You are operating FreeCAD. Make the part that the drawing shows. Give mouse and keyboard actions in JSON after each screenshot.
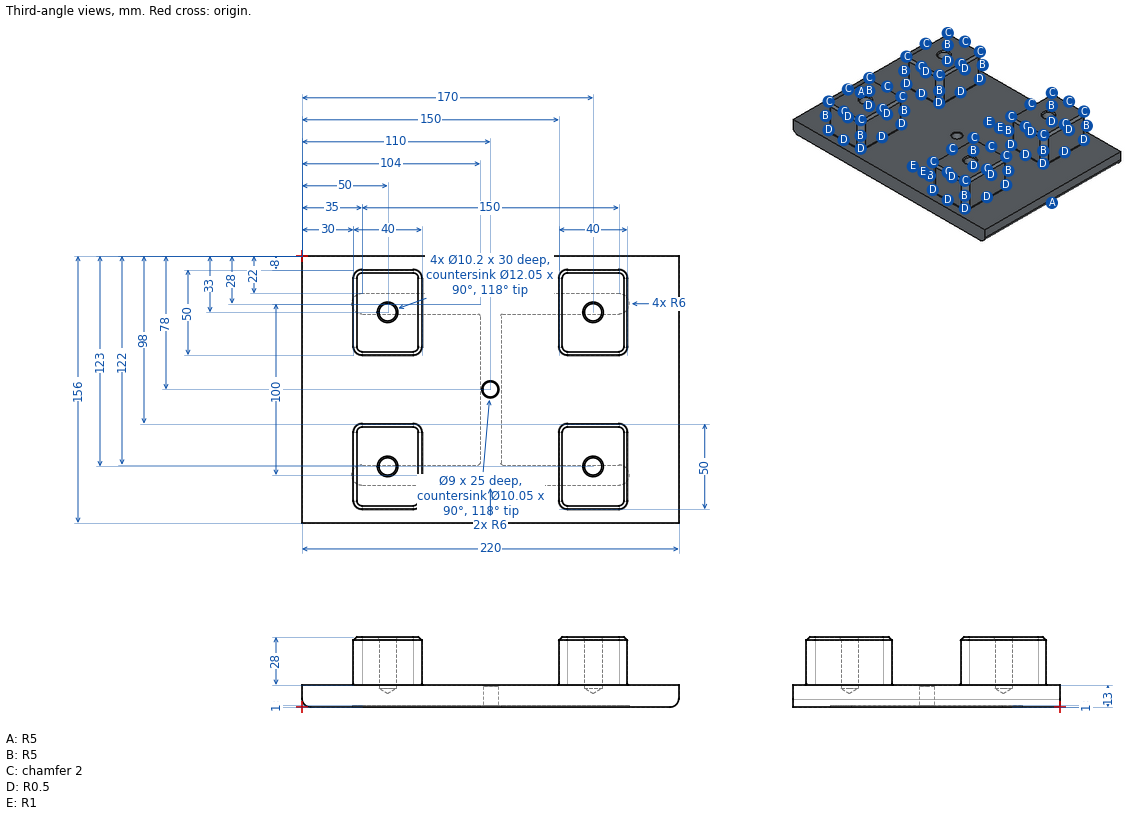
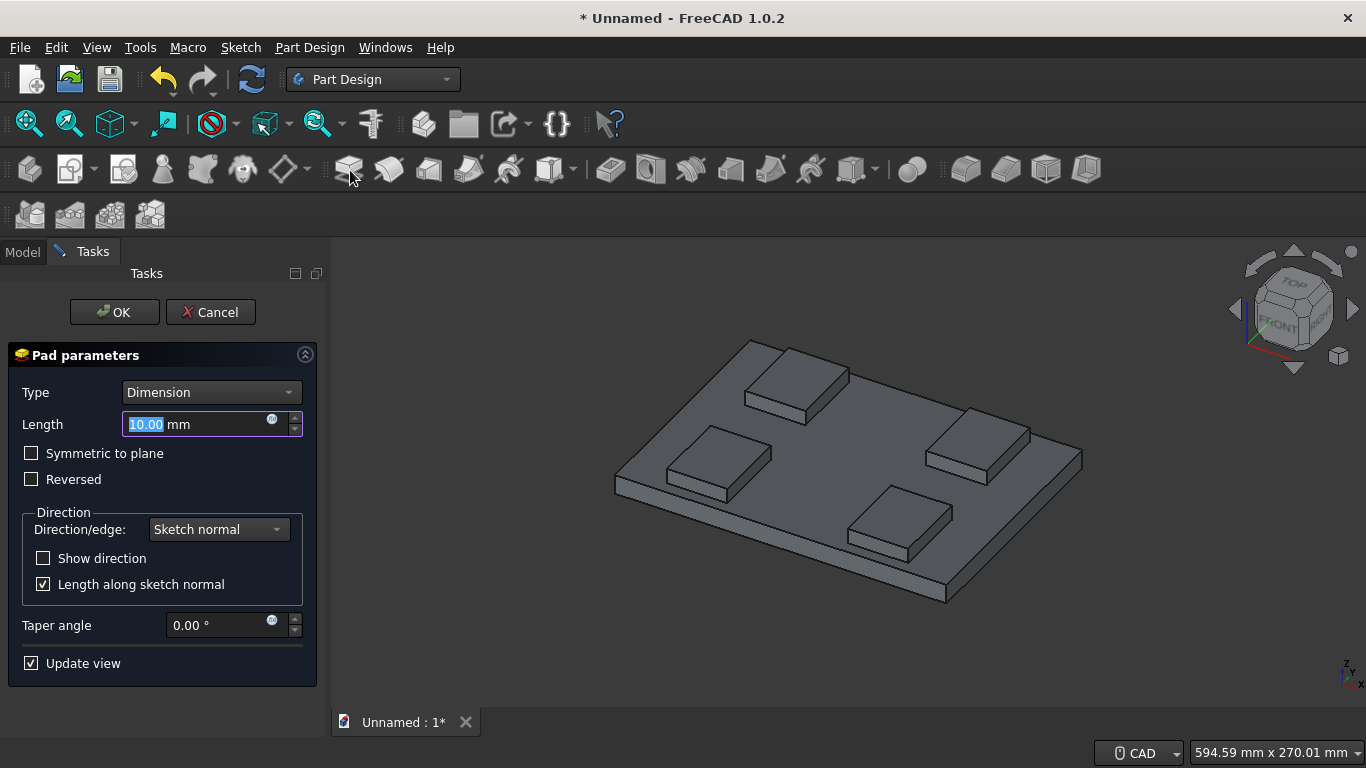
{"action": "type", "text": "28"}
{"action": "key", "text": "Tab"}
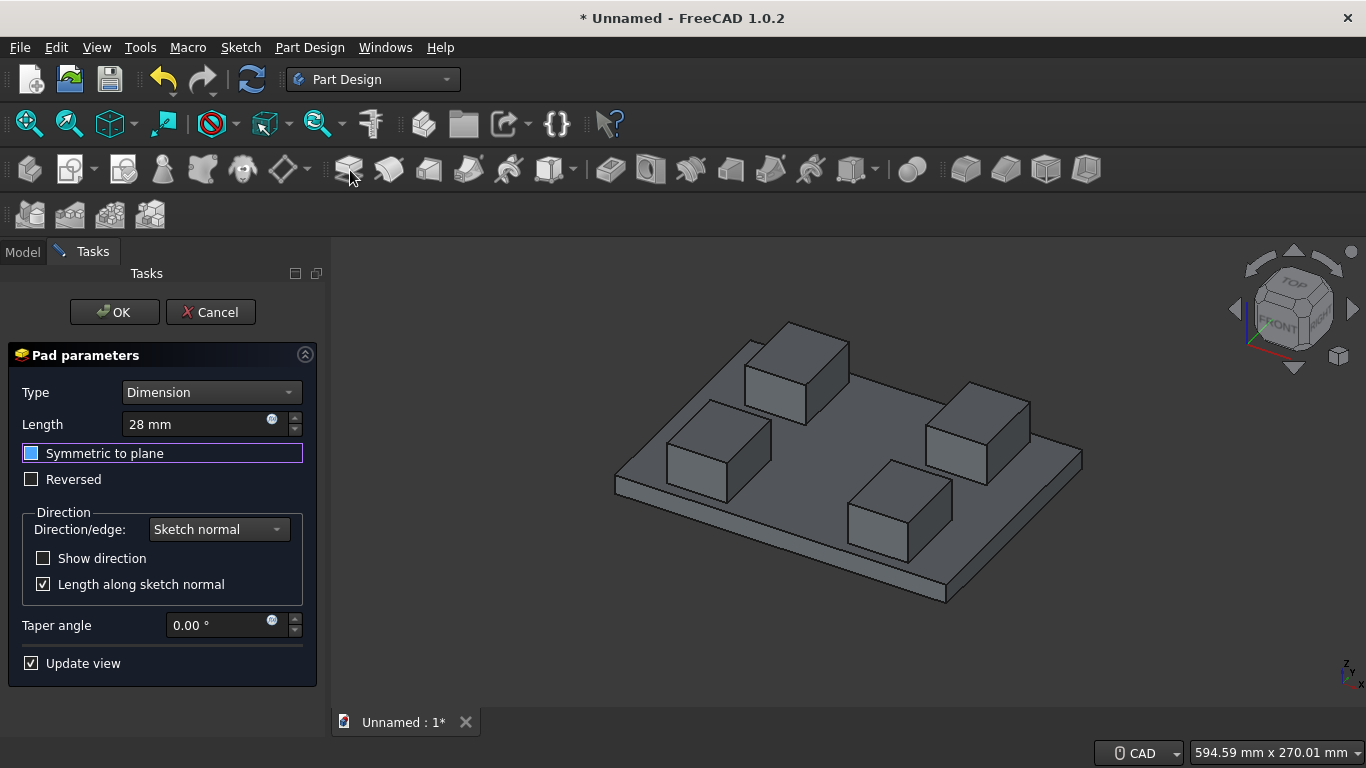
{"action": "left_click", "coordinate": [115, 312]}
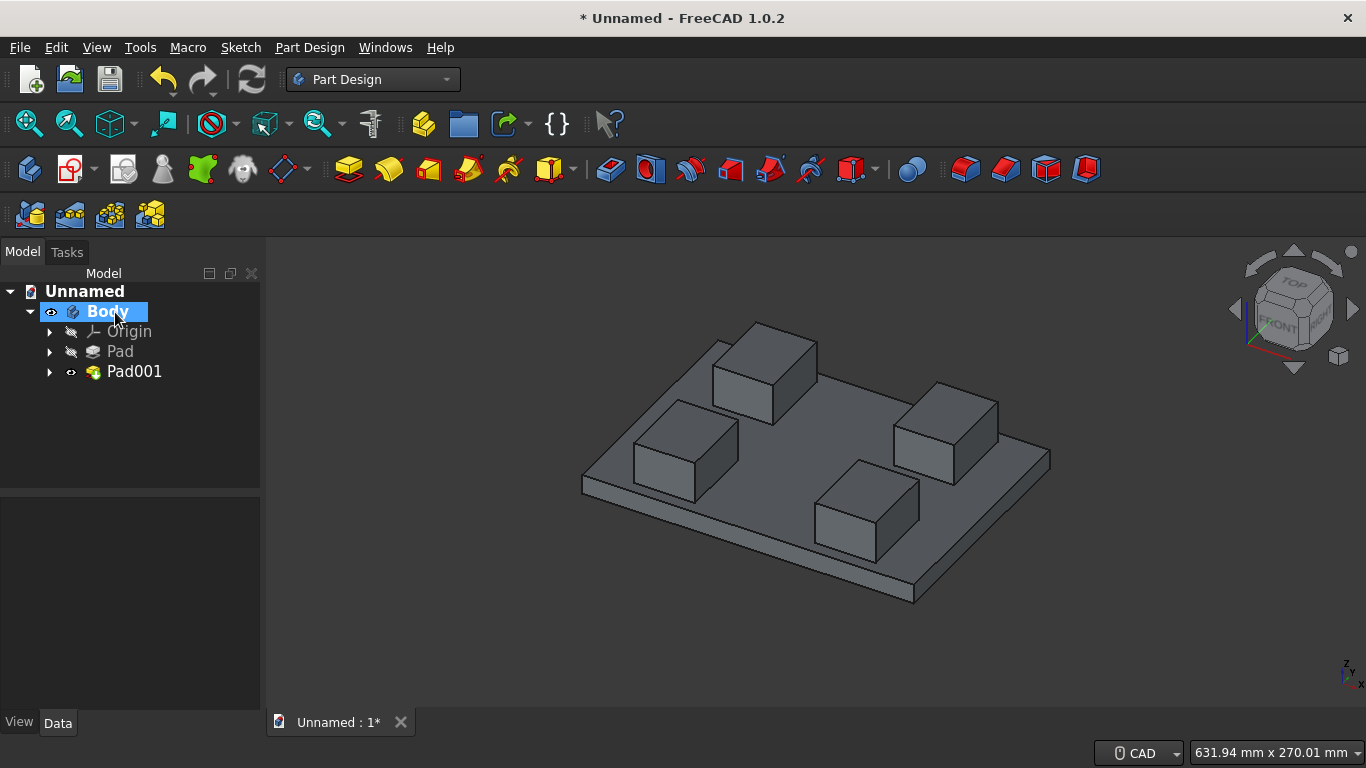
{"action": "key", "text": "0"}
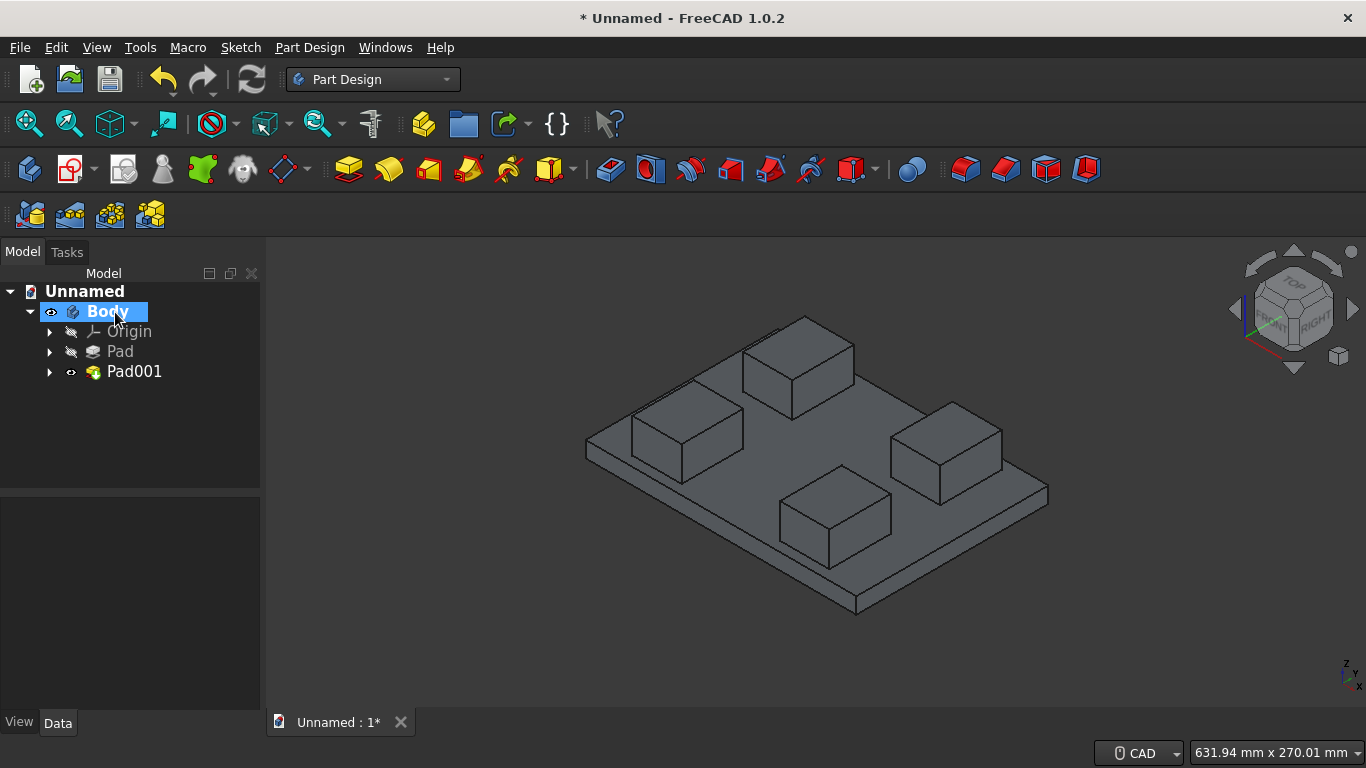
{"action": "key", "text": "2"}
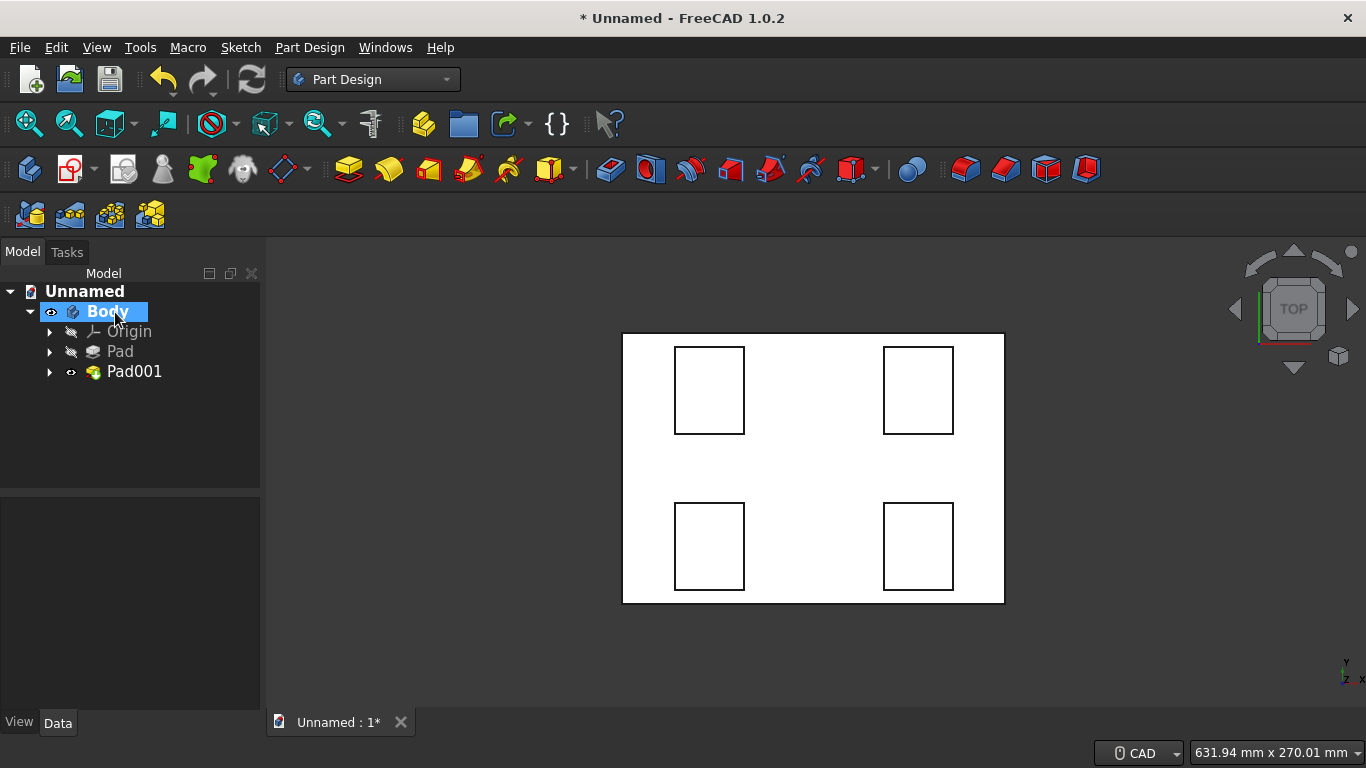
{"action": "key", "text": "1"}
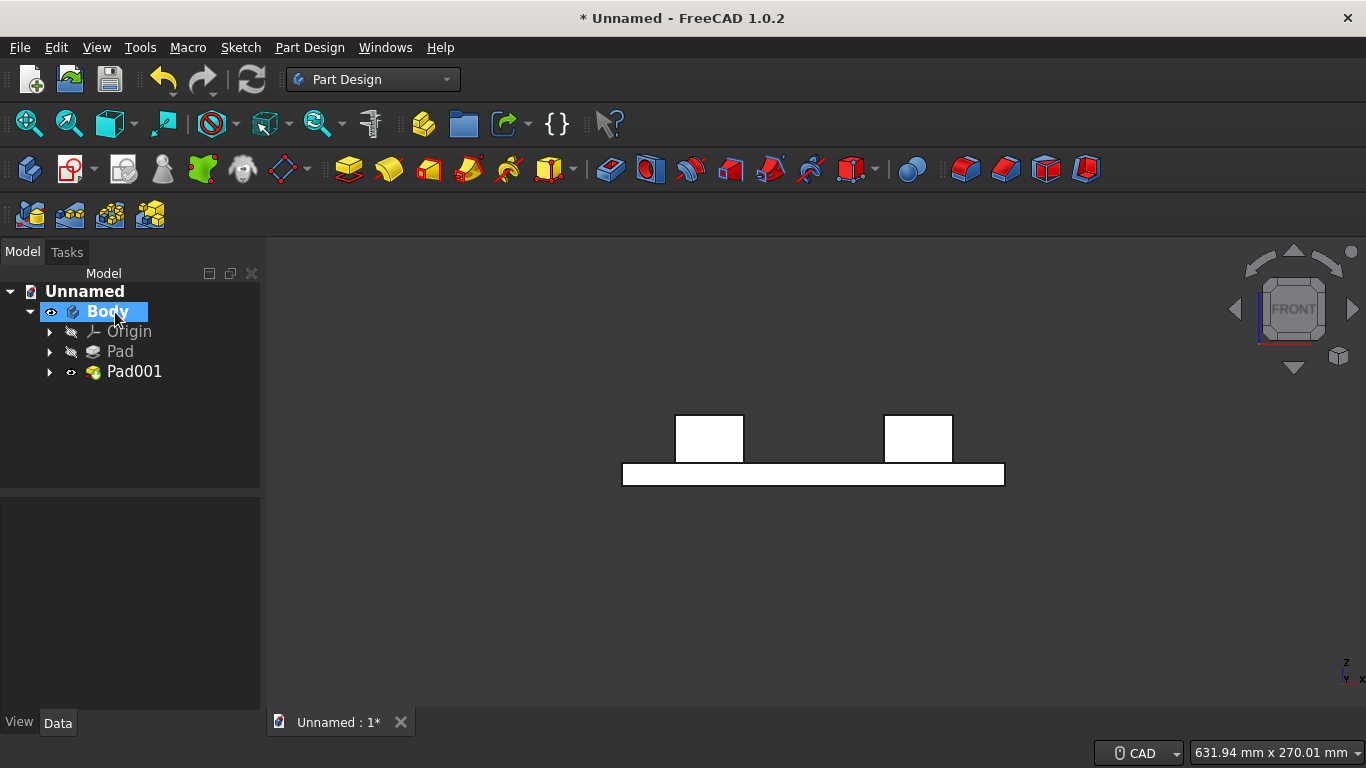
{"action": "left_click", "coordinate": [30, 124]}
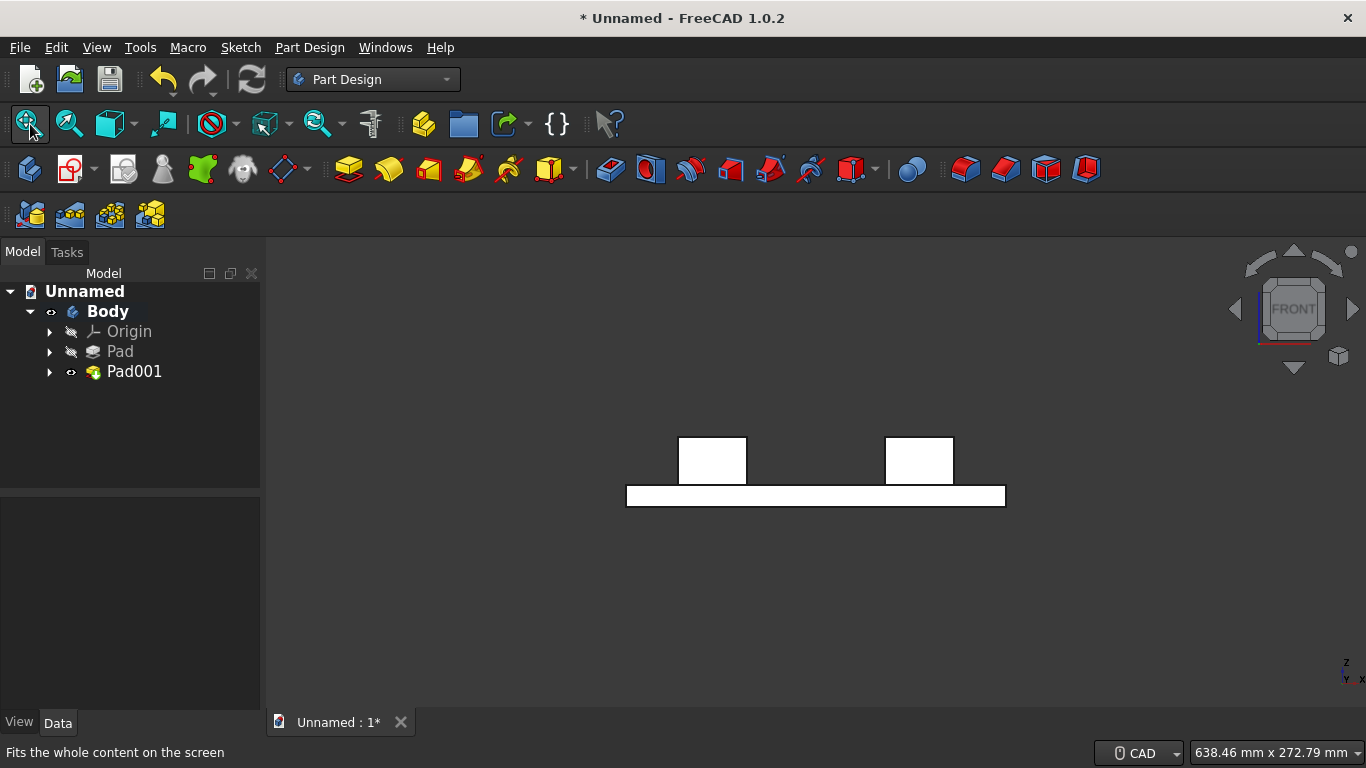
{"action": "key", "text": "3"}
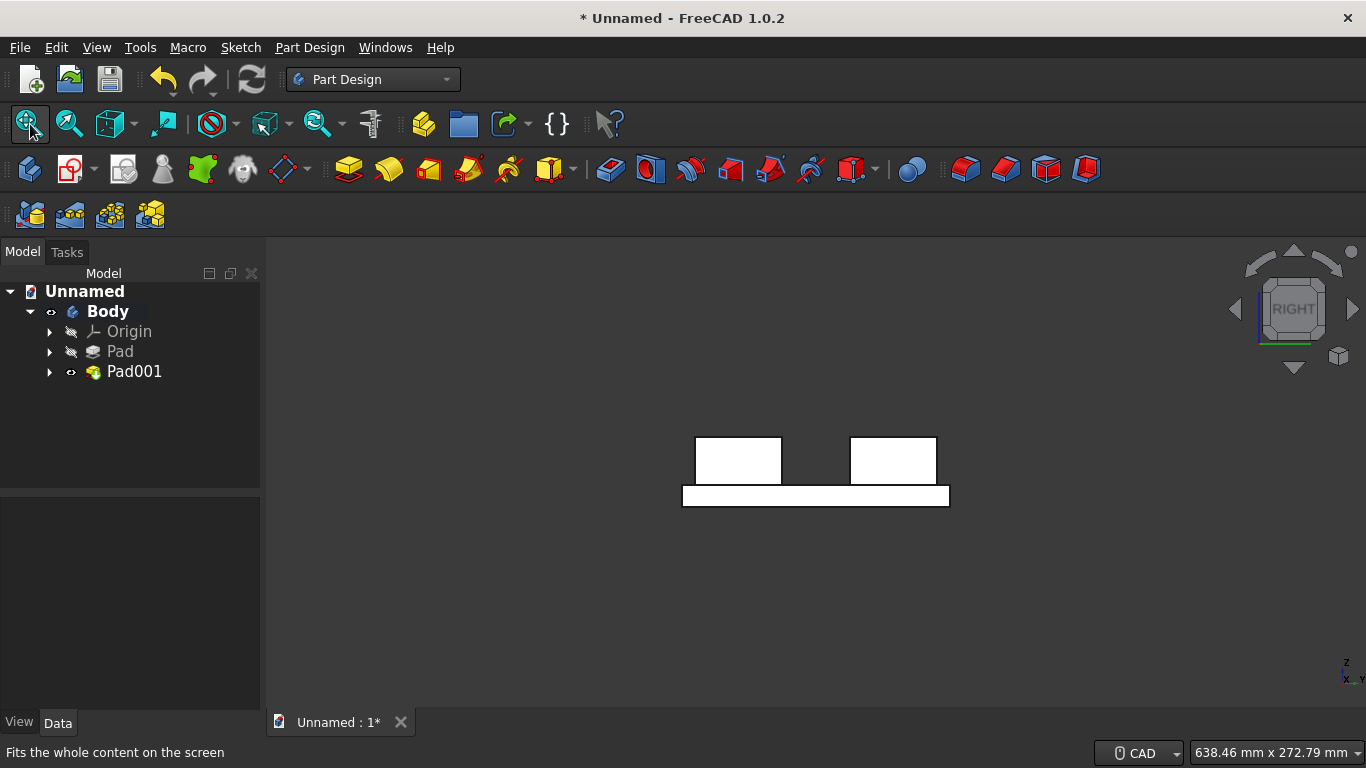
{"action": "key", "text": "v f"}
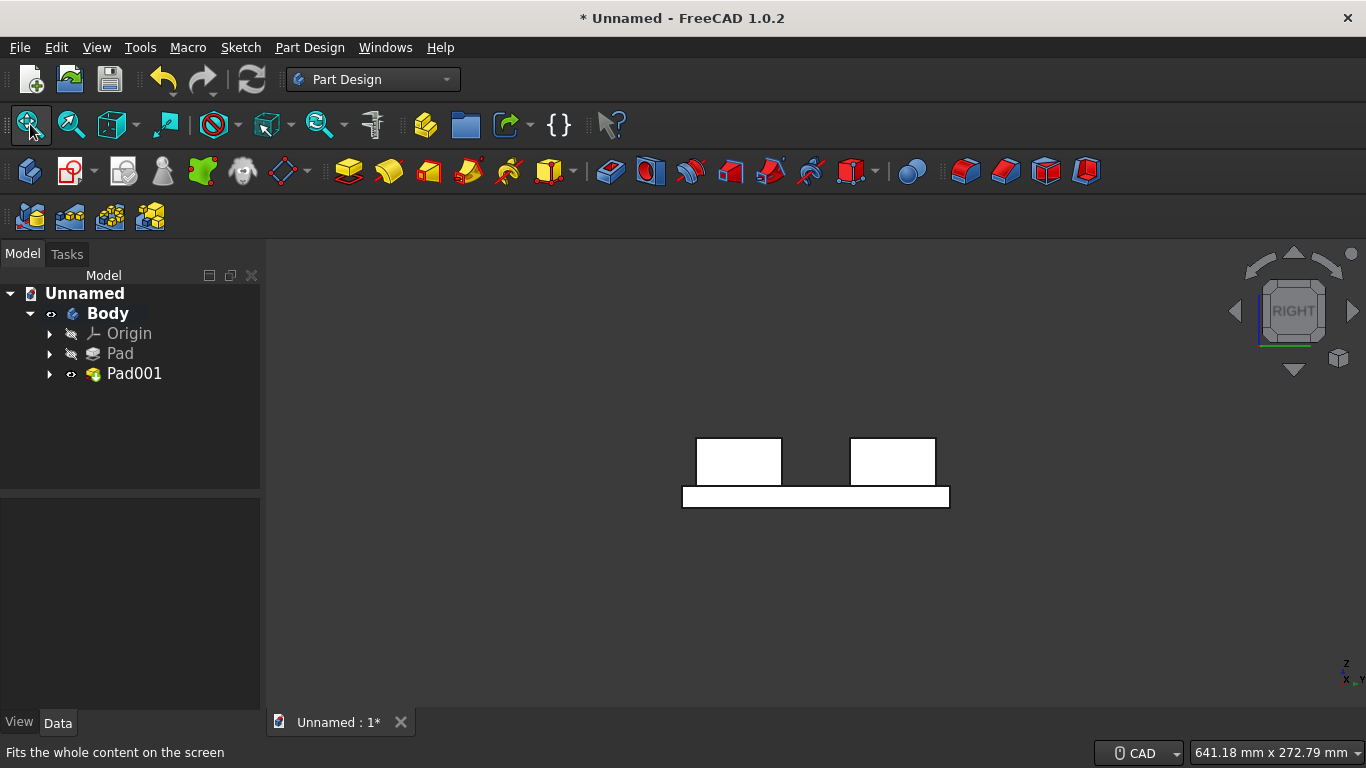
{"action": "left_click", "coordinate": [816, 507]}